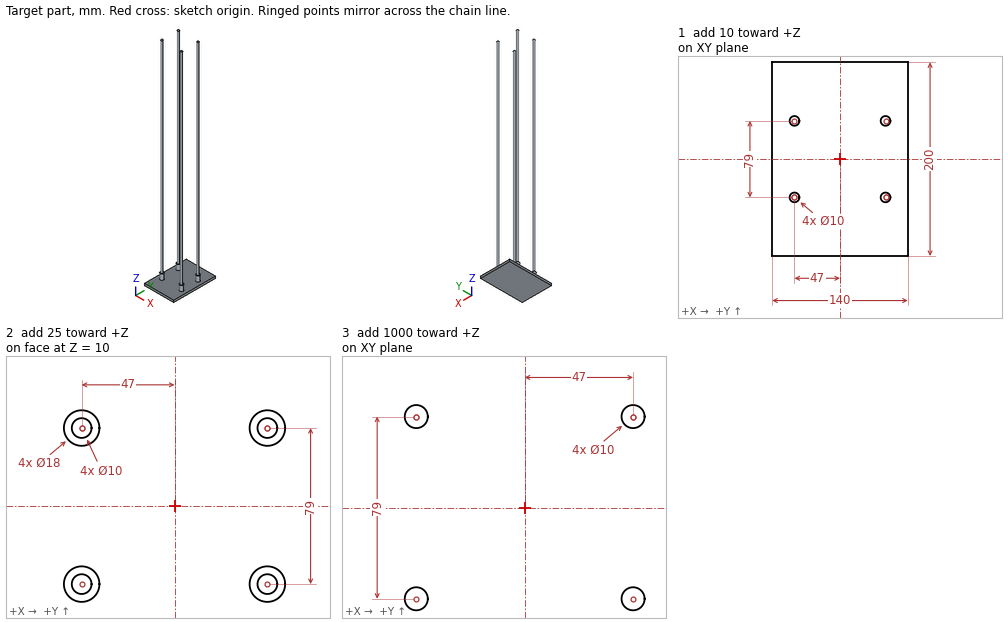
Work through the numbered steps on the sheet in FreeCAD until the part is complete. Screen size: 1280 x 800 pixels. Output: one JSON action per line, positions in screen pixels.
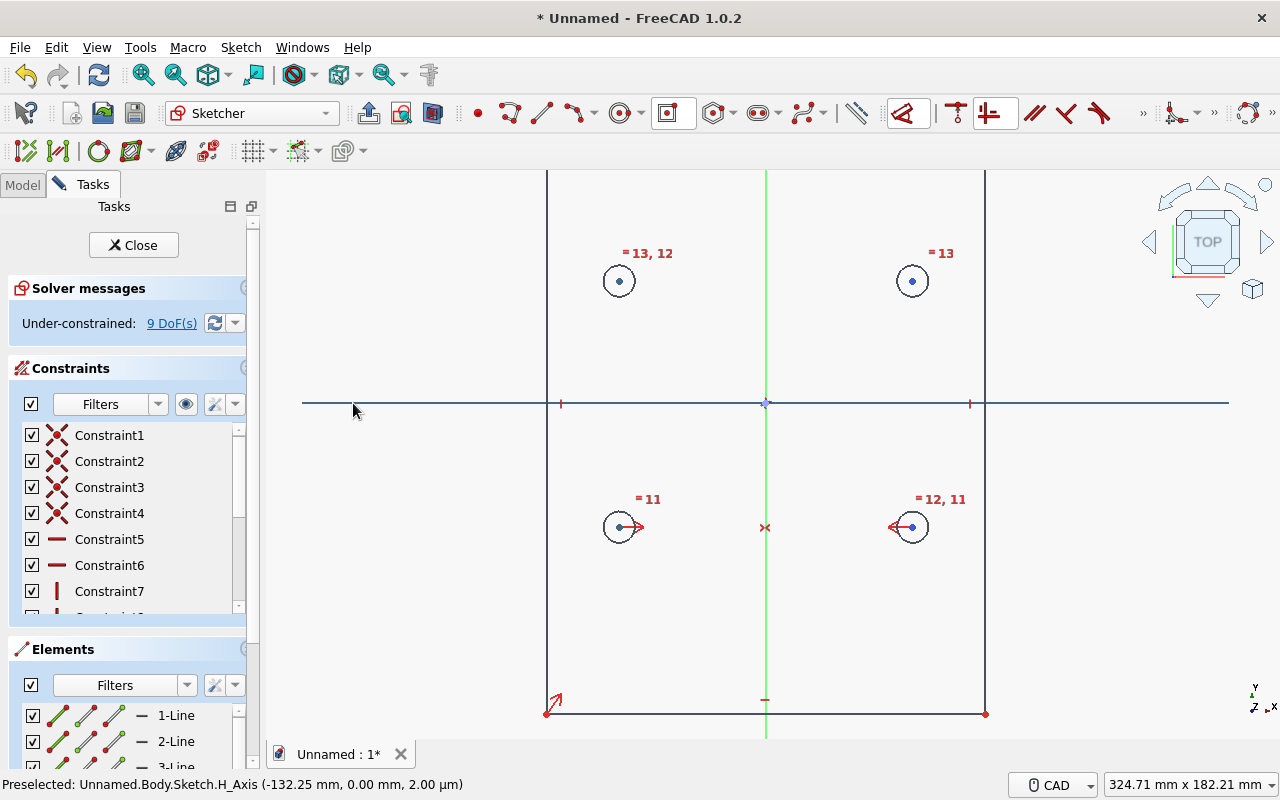
{"action": "key", "text": "s"}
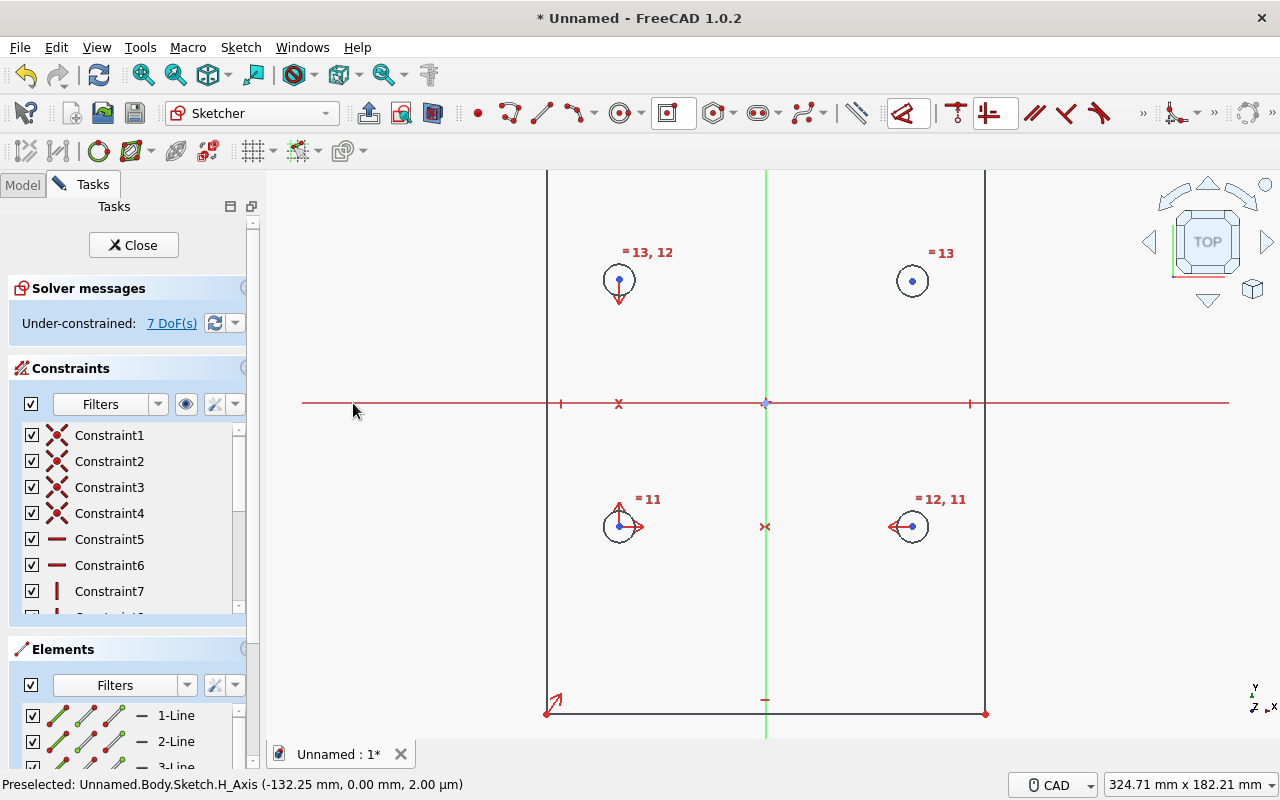
{"action": "left_click", "coordinate": [913, 527]}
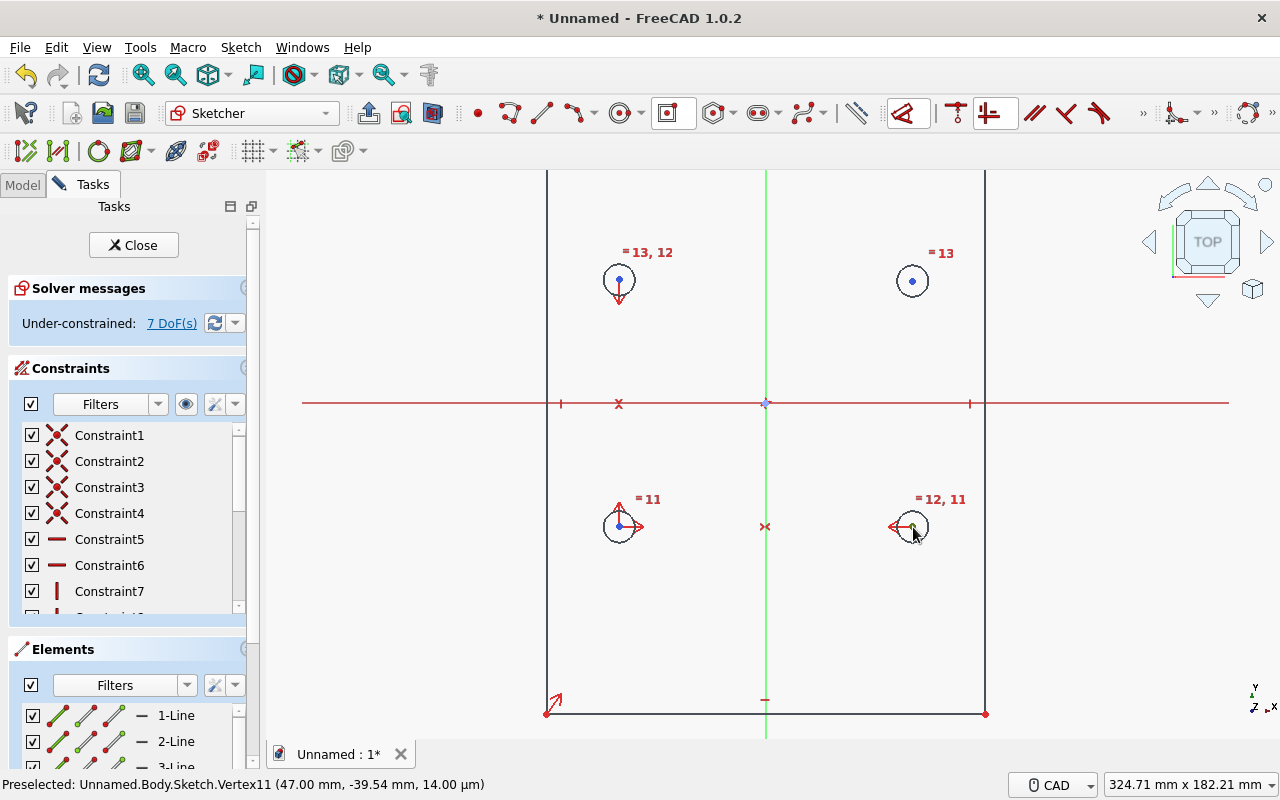
{"action": "left_click", "coordinate": [913, 281]}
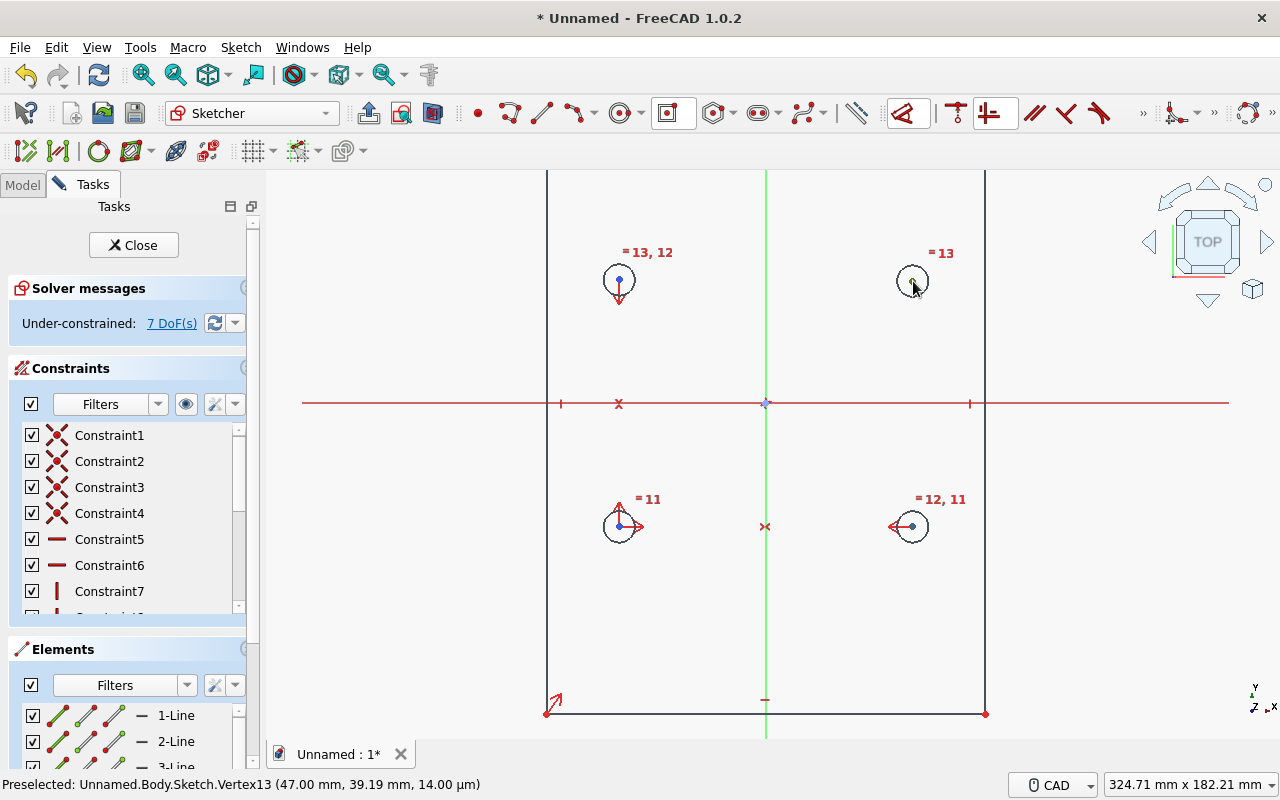
{"action": "left_click", "coordinate": [353, 403]}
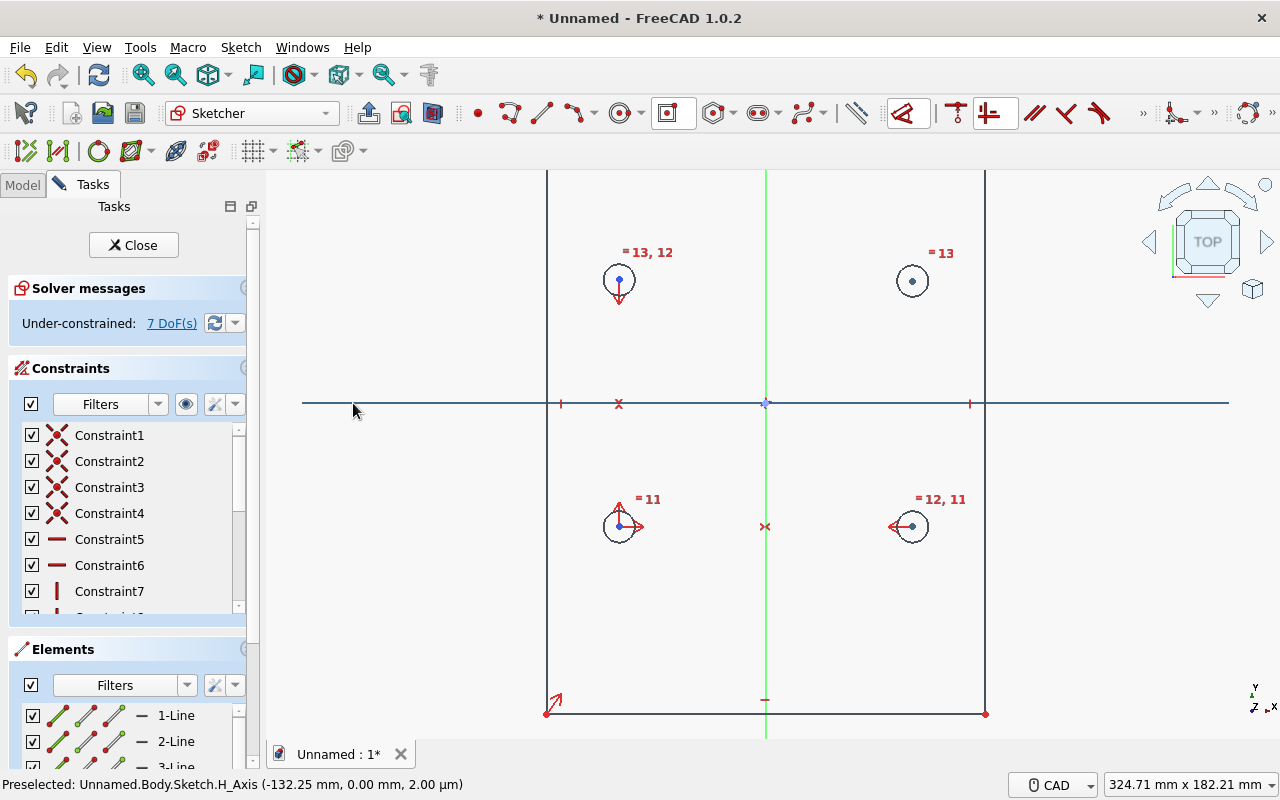
{"action": "key", "text": "s"}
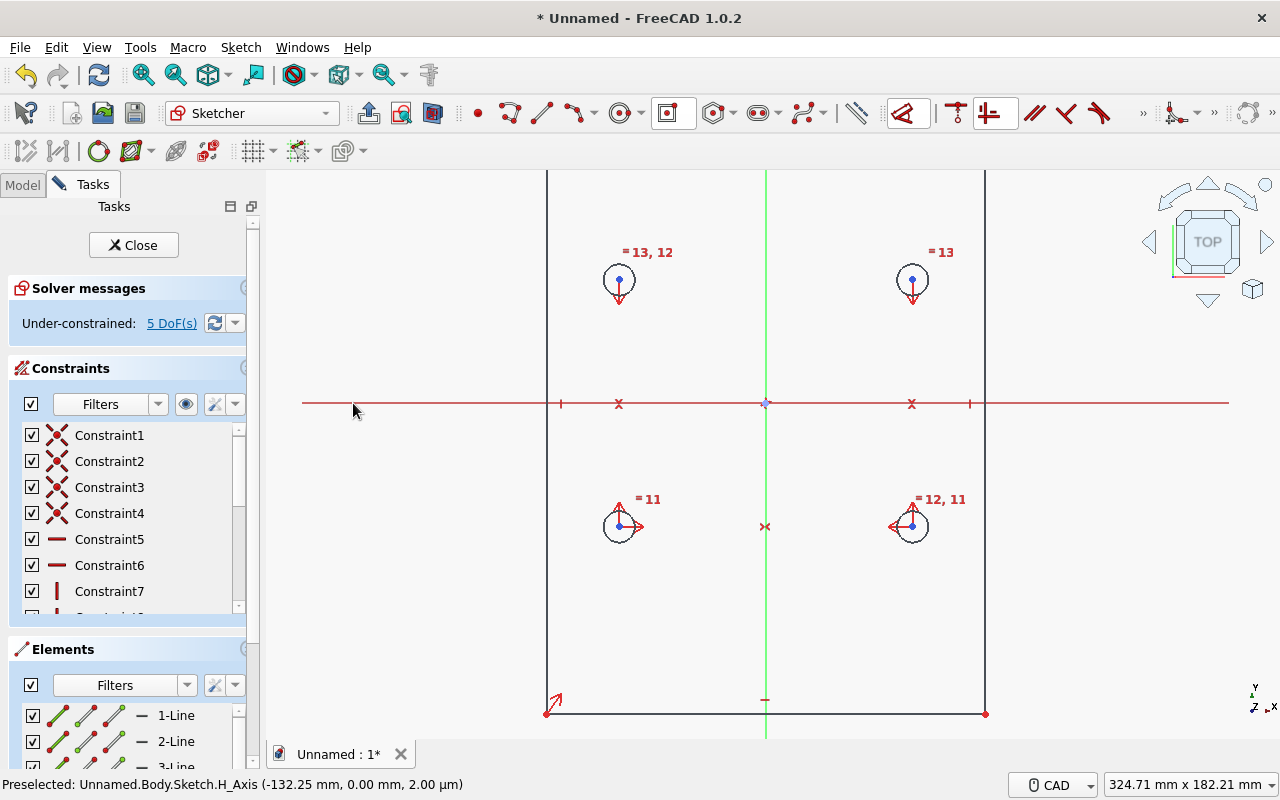
{"action": "left_click", "coordinate": [902, 114]}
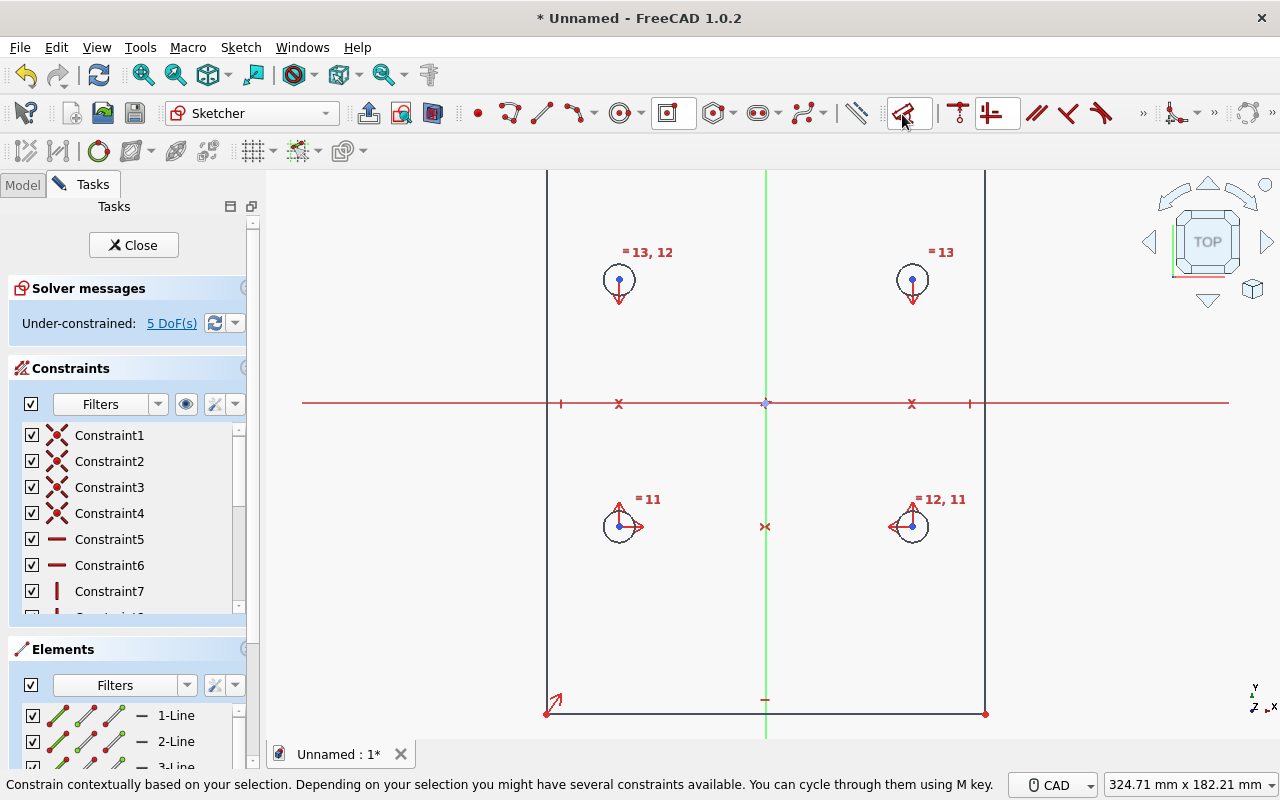
{"action": "scroll", "coordinate": [630, 516], "scroll_direction": "up", "scroll_amount": 2}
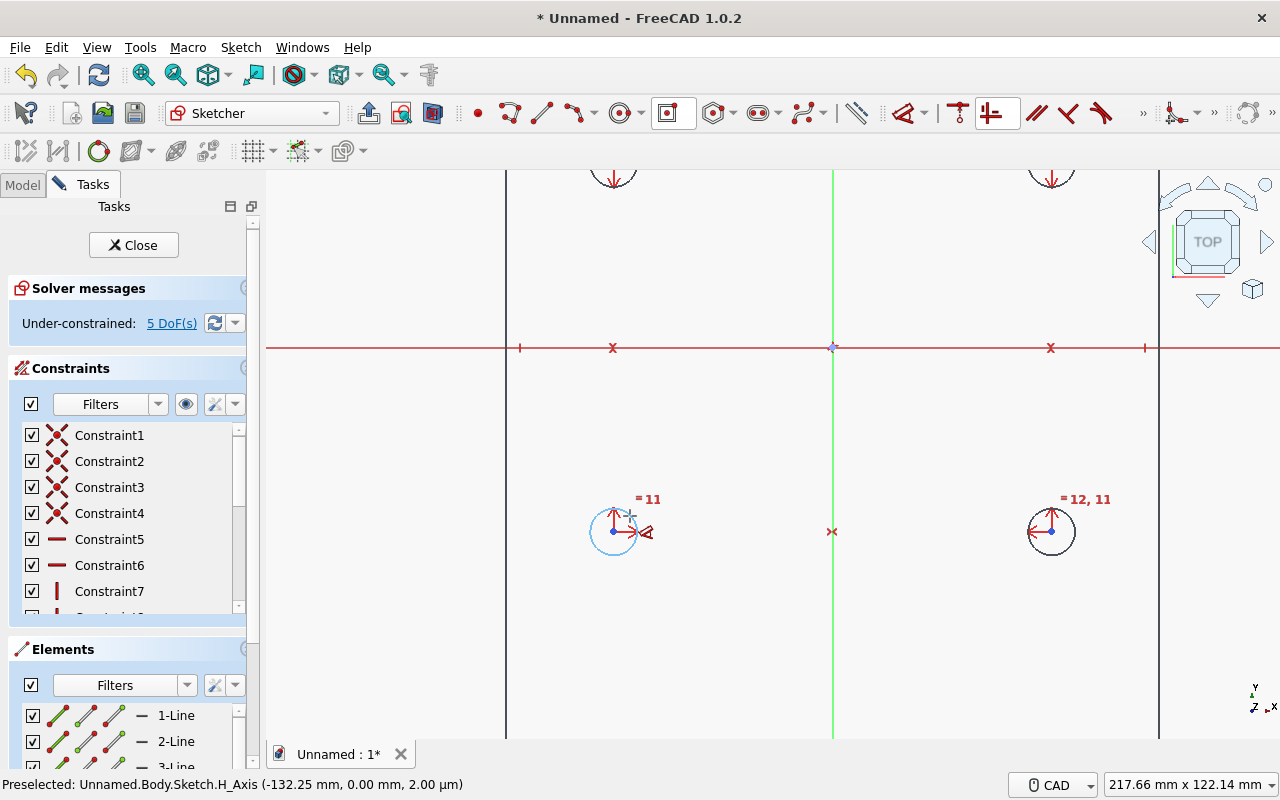
{"action": "left_click", "coordinate": [630, 515]}
{"action": "left_click", "coordinate": [652, 492]}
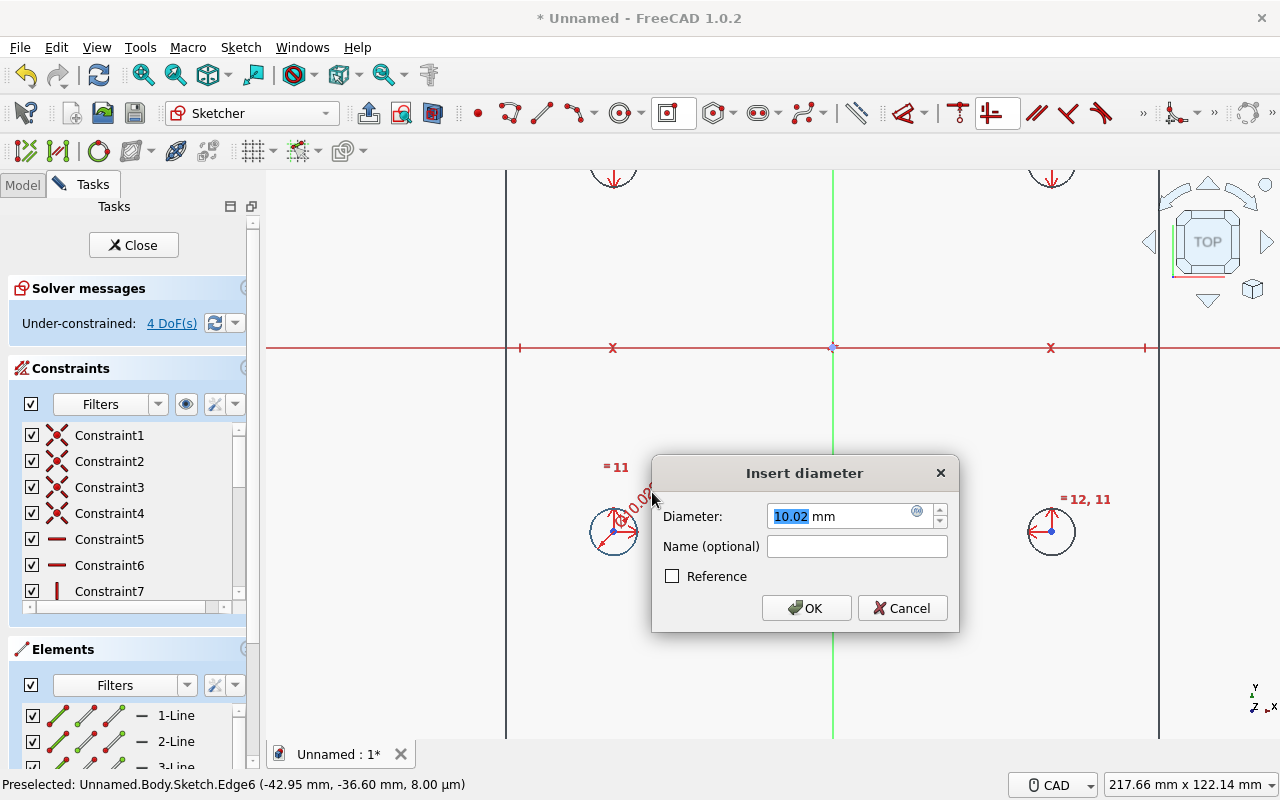
{"action": "type", "text": "10"}
{"action": "key", "text": "Return"}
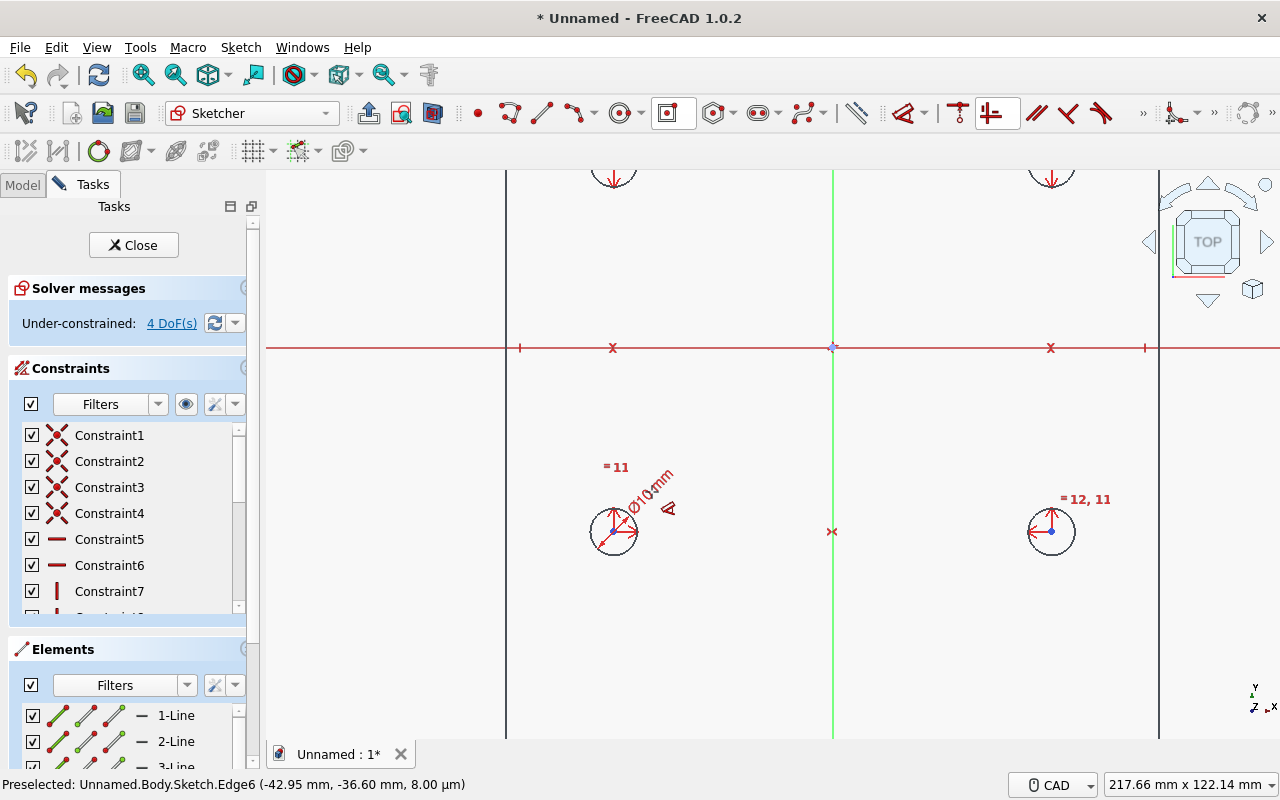
{"action": "left_click", "coordinate": [614, 532]}
{"action": "left_click", "coordinate": [723, 566]}